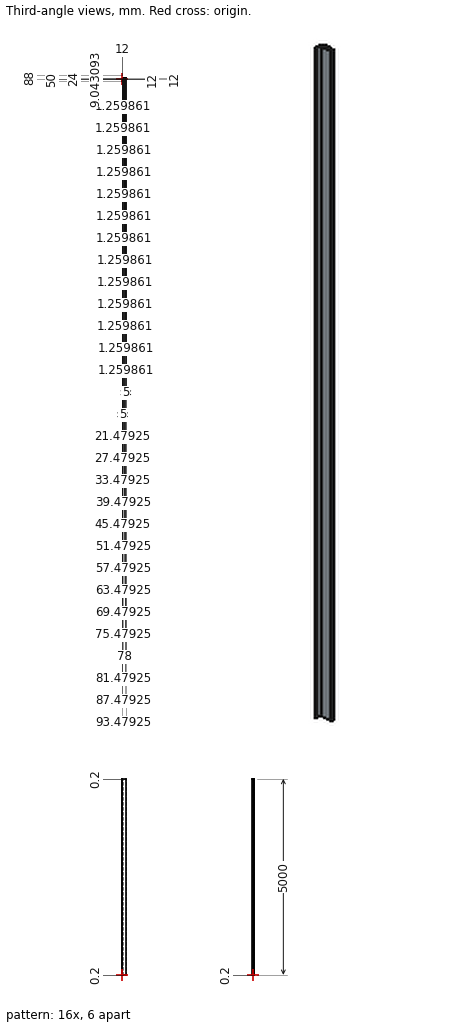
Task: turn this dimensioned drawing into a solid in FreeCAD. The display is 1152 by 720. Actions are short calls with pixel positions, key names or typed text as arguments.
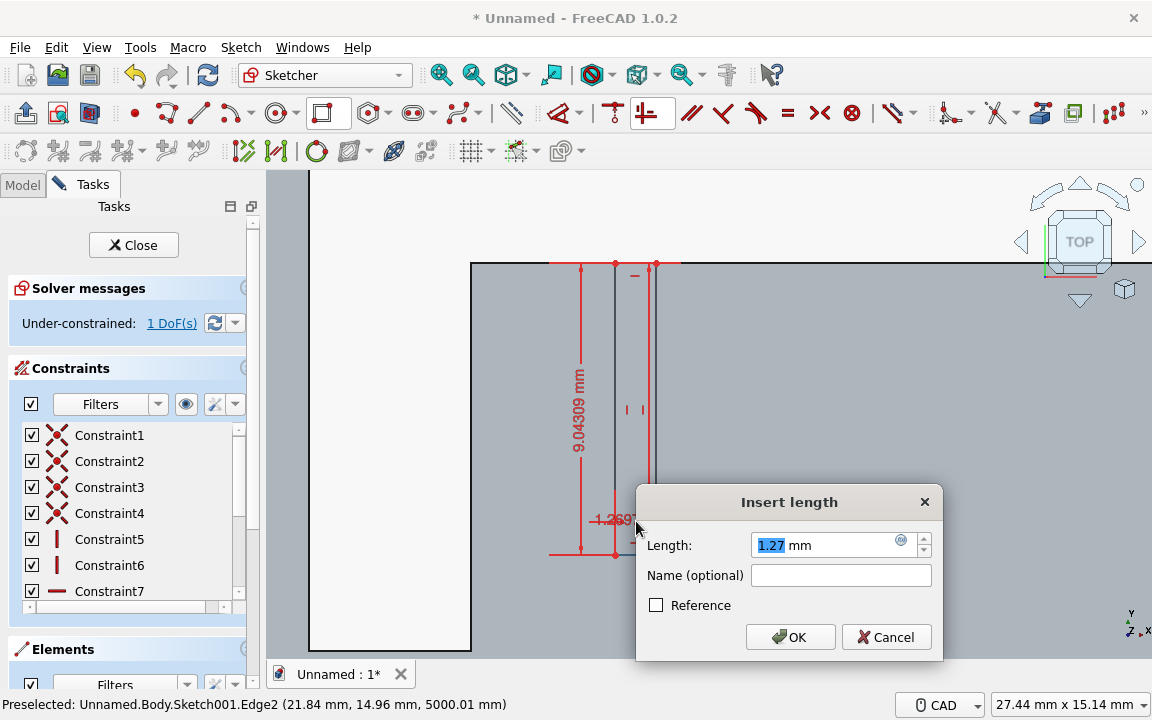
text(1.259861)
key(Return)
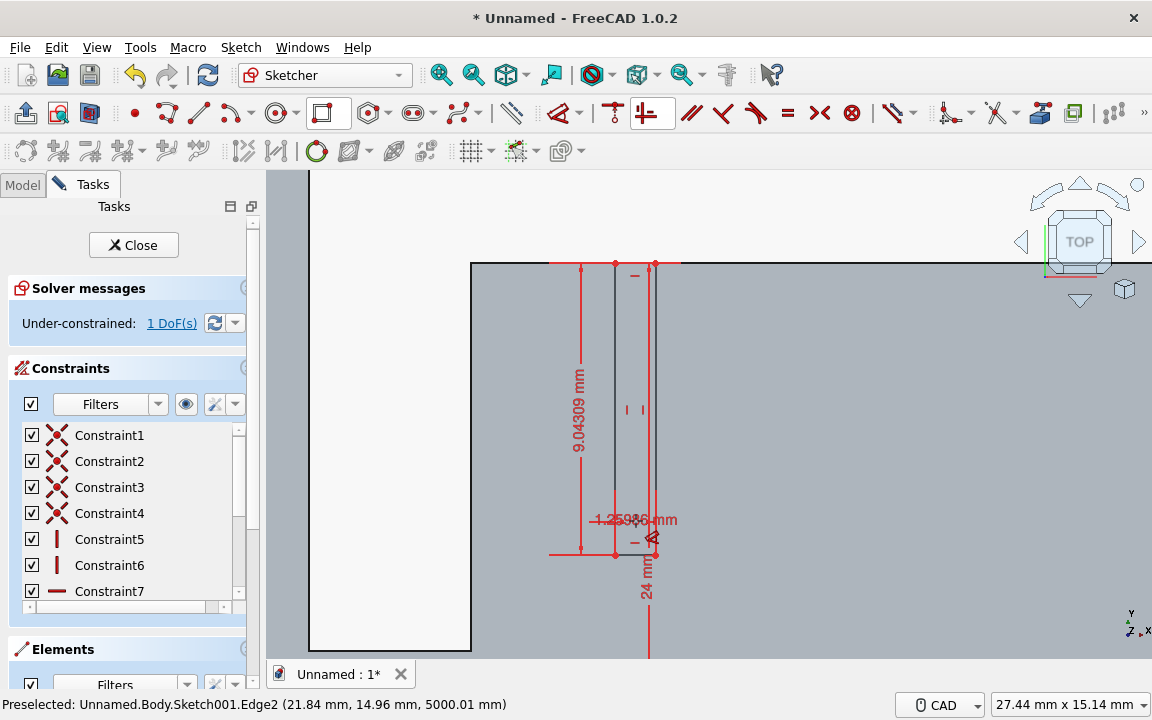
click(615, 263)
click(454, 229)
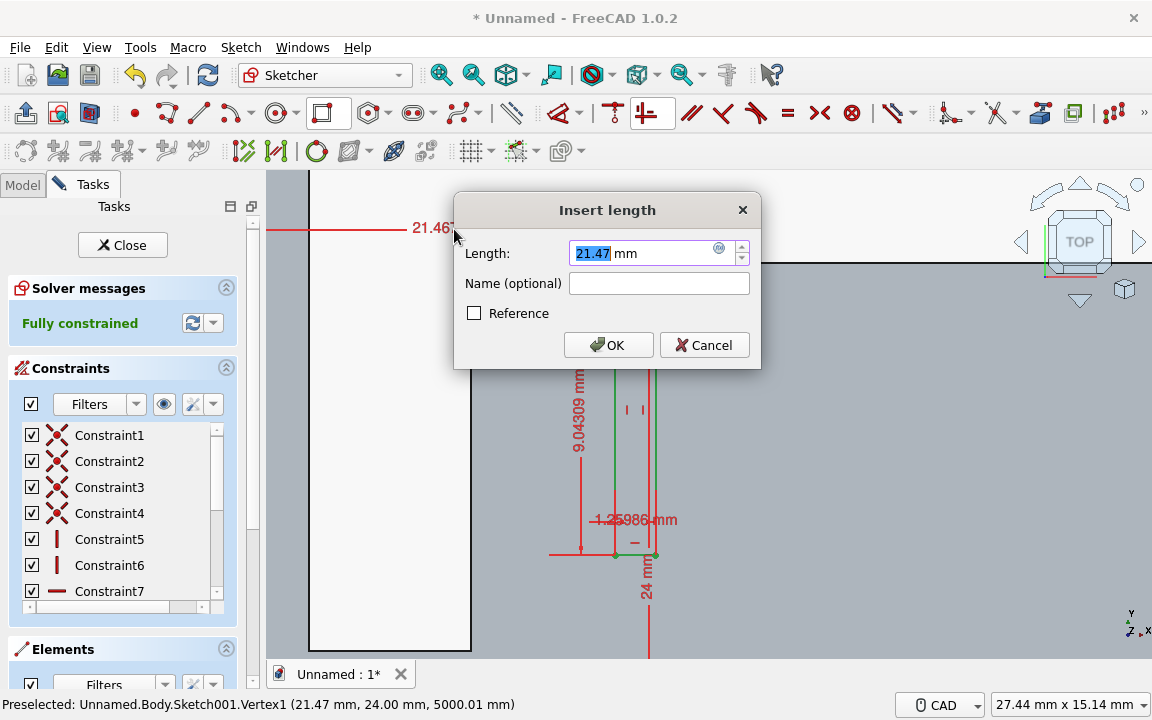
text(21.47925)
key(Return)
key(Escape)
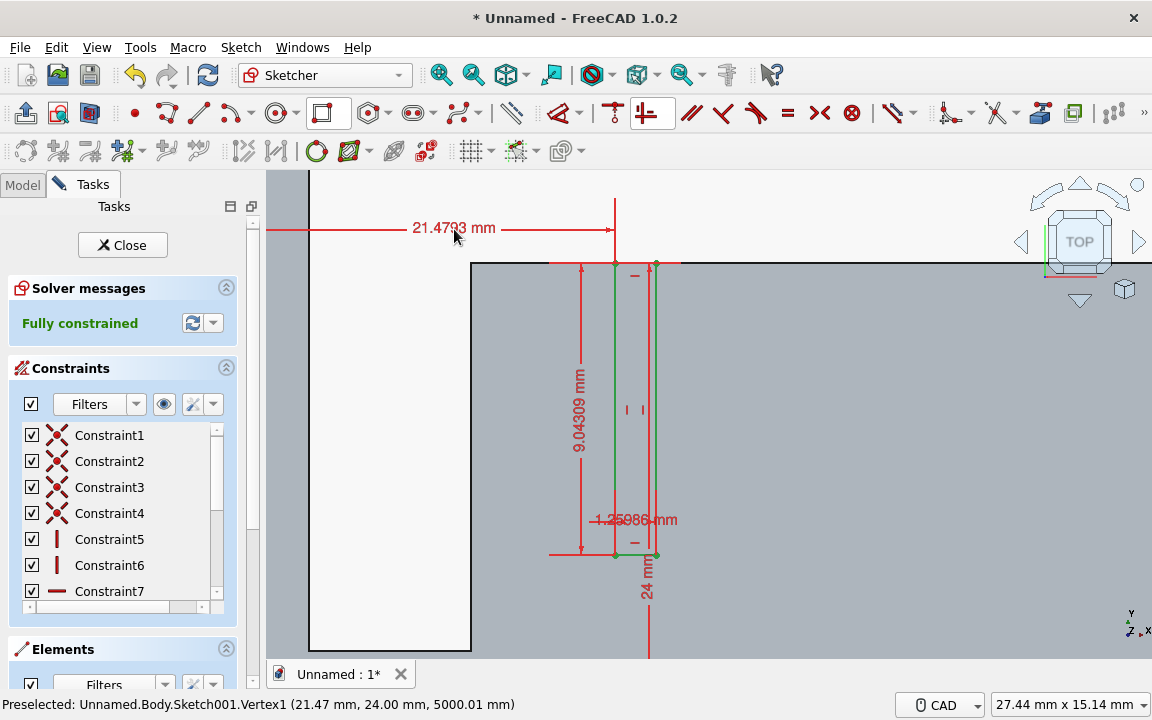
click(123, 245)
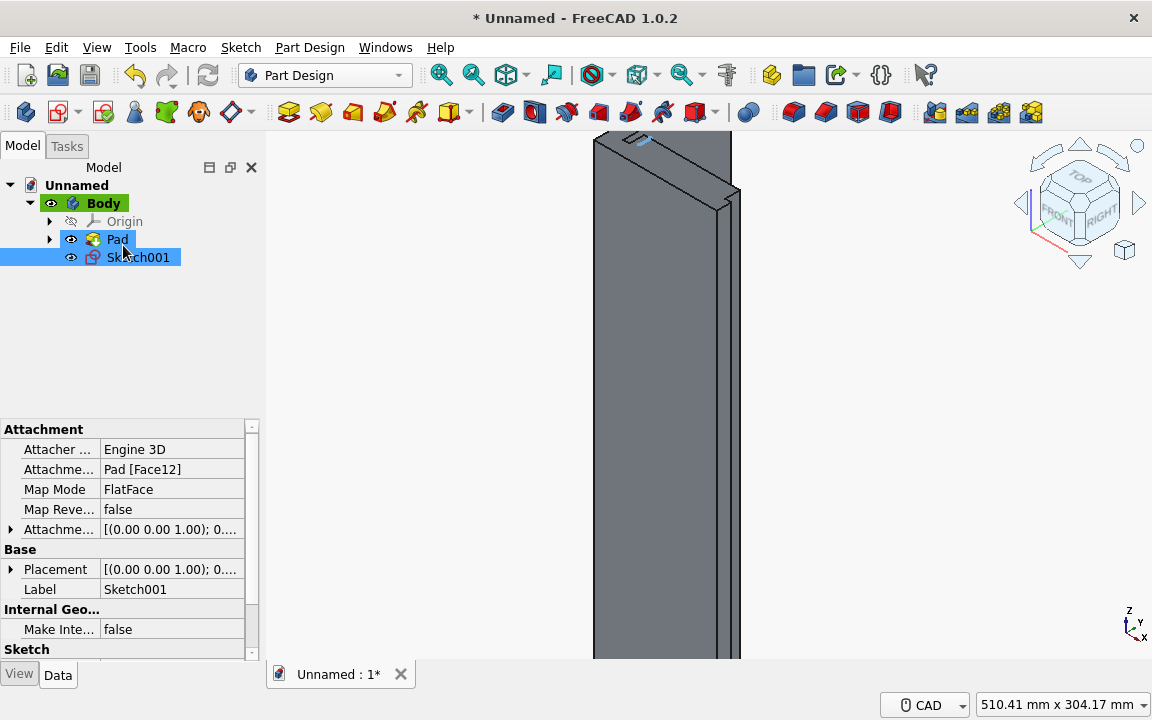
click(504, 112)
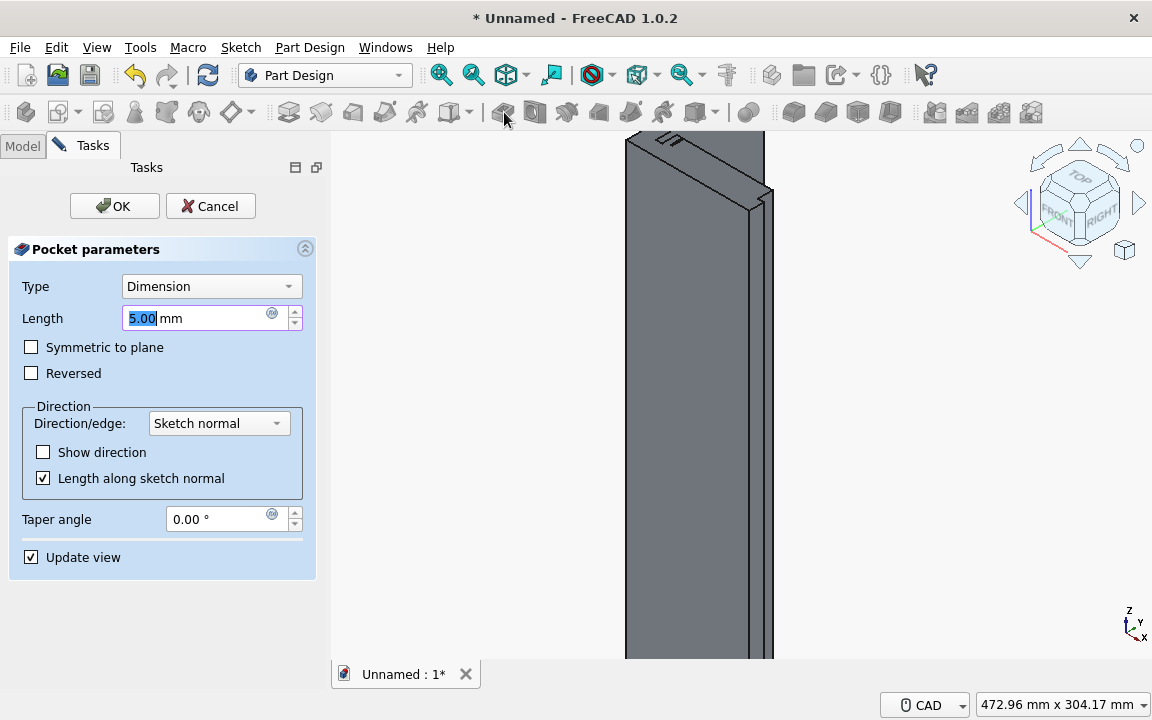
text(0.2)
key(Tab)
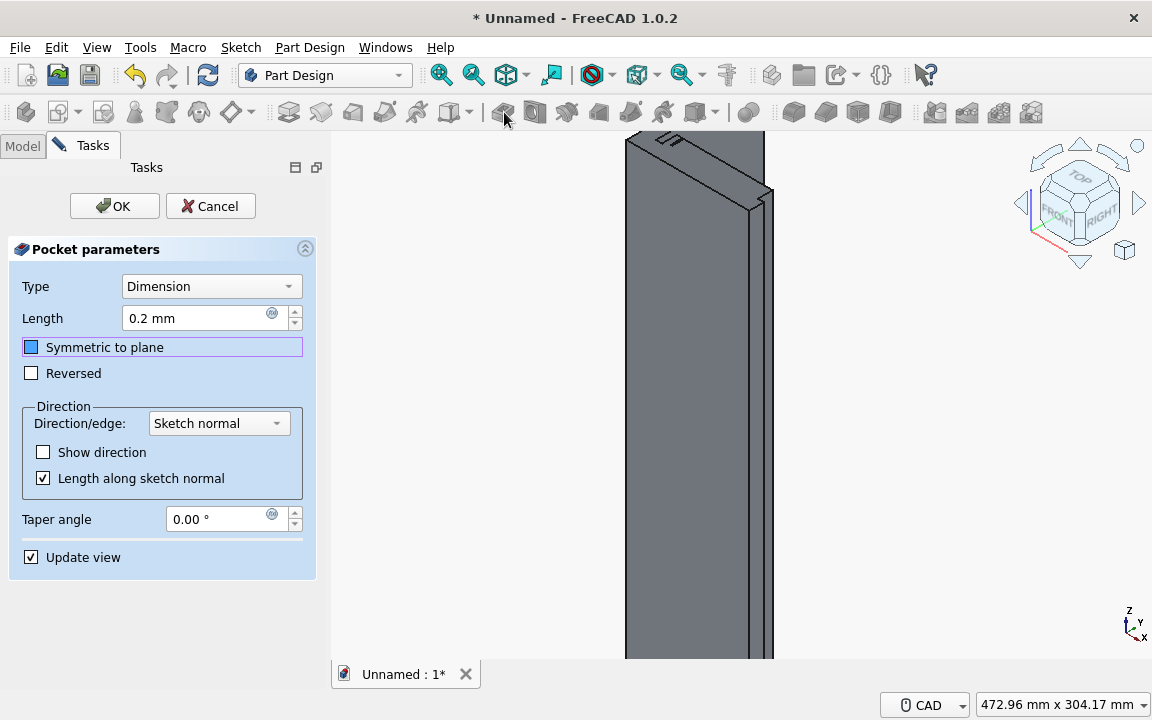
click(115, 206)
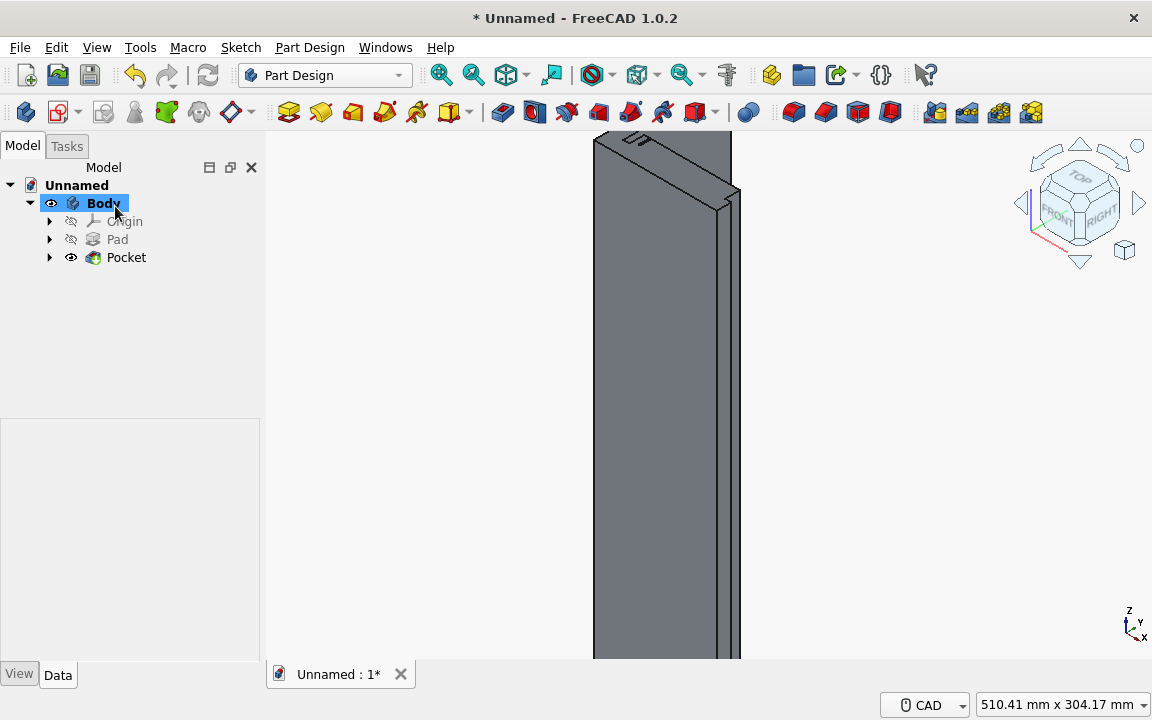
click(442, 76)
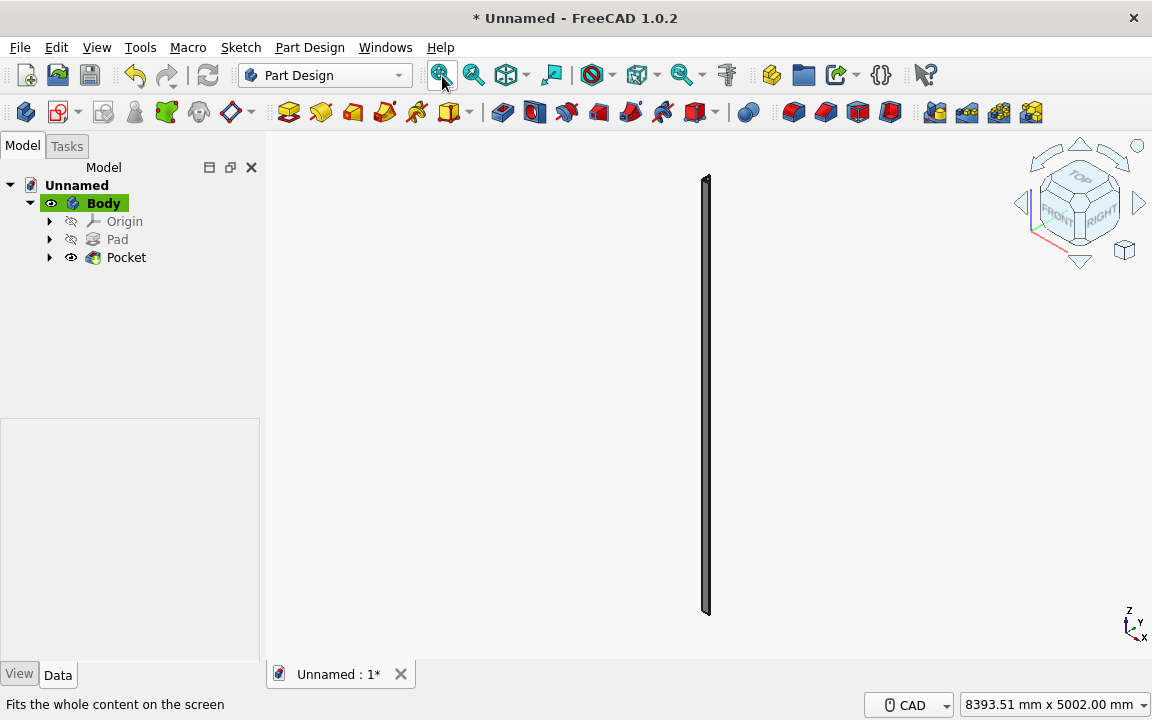
click(116, 257)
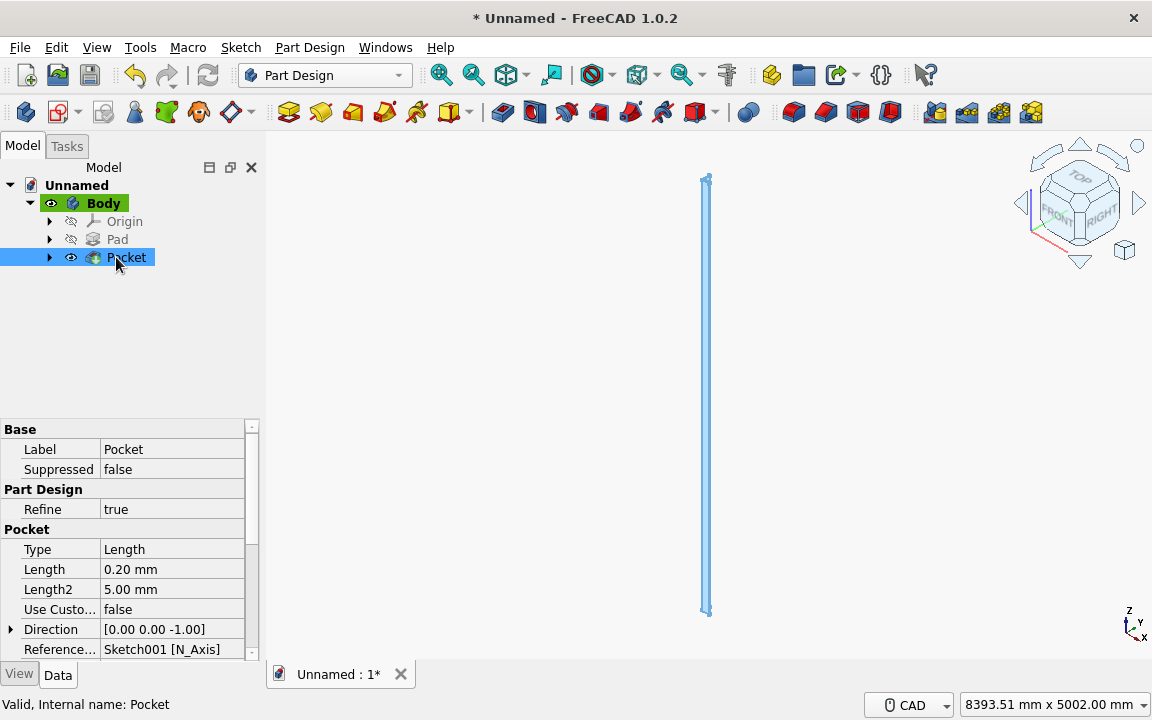
click(968, 112)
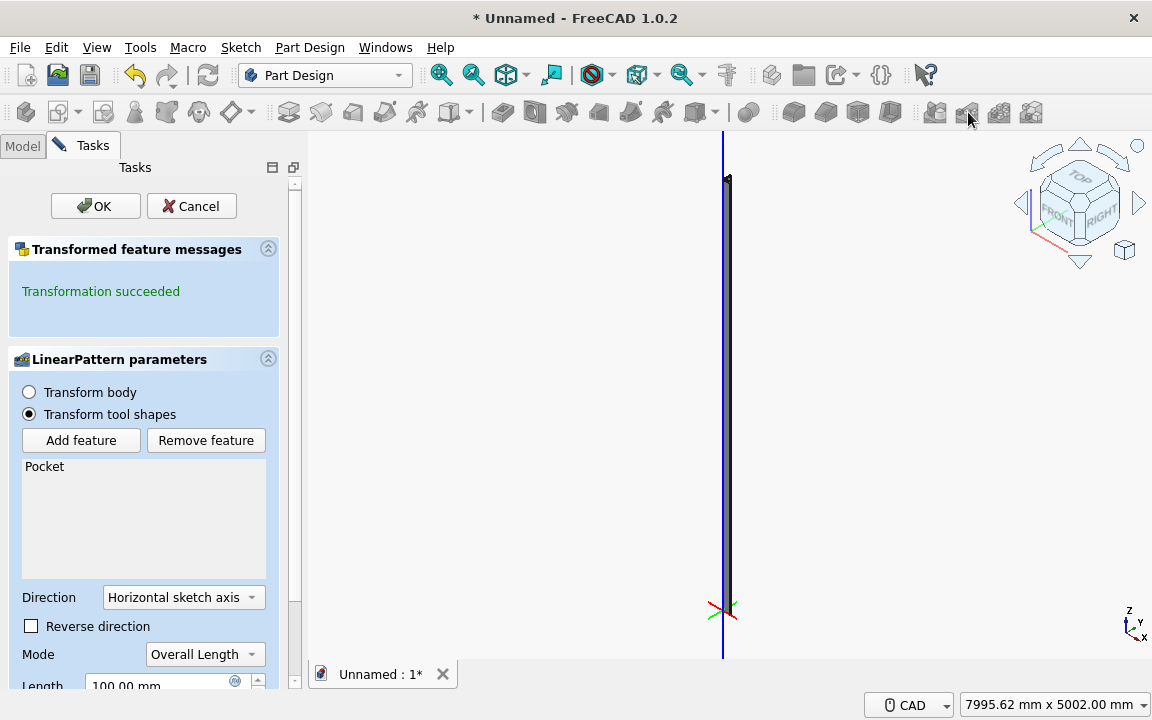
click(184, 598)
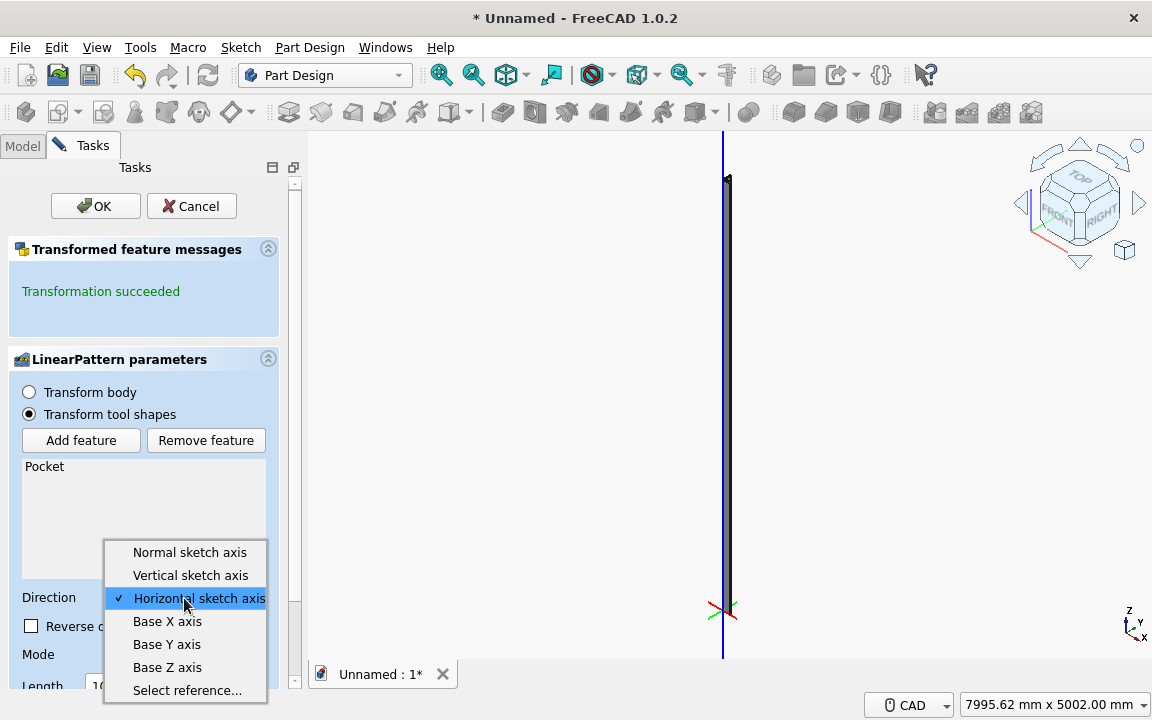
click(184, 622)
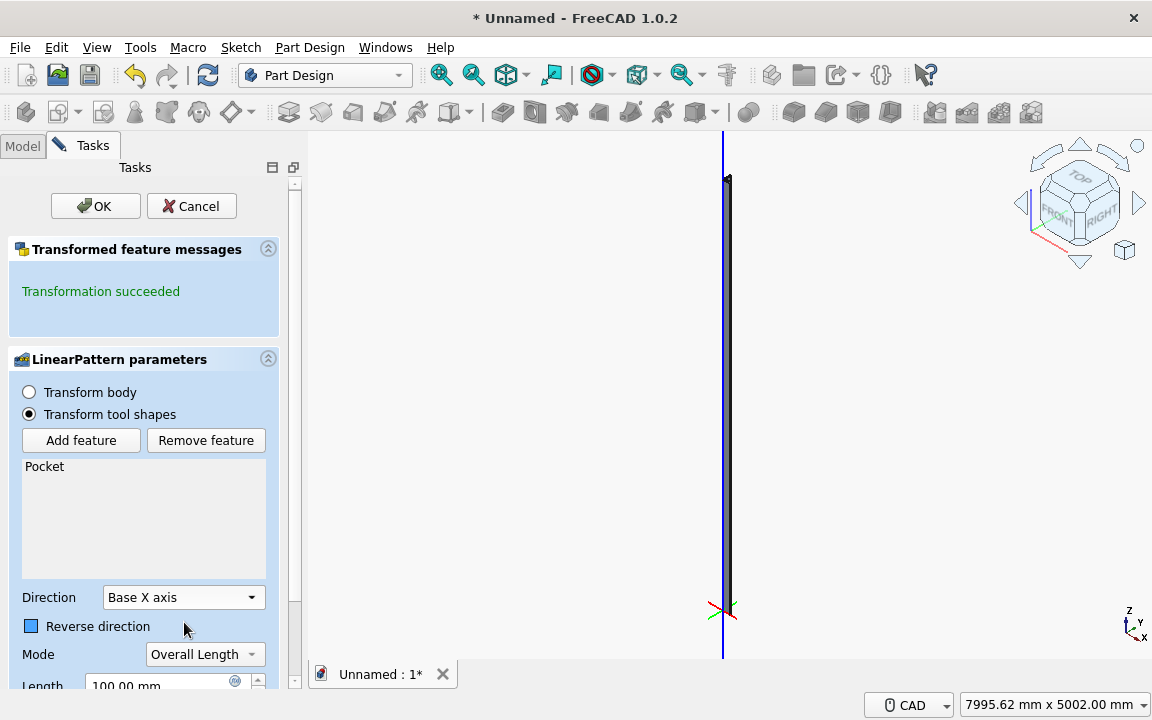
click(206, 654)